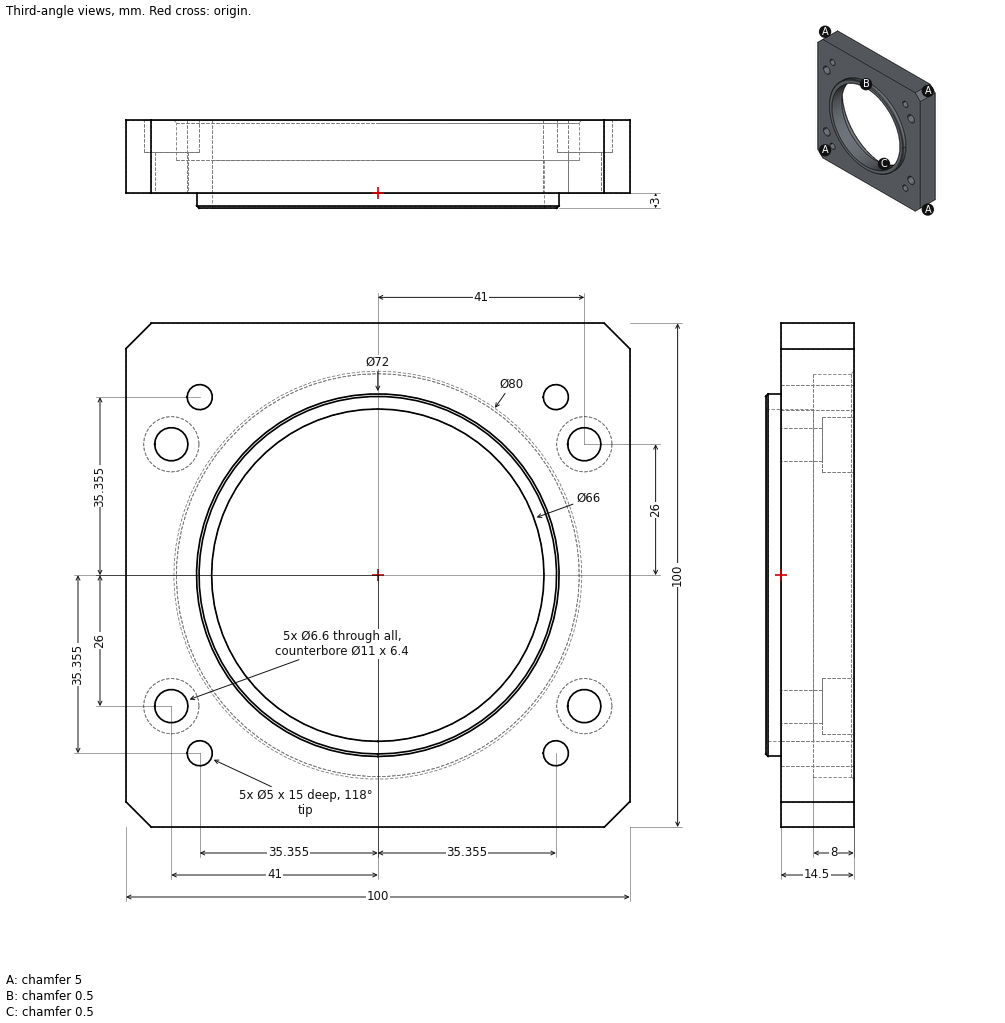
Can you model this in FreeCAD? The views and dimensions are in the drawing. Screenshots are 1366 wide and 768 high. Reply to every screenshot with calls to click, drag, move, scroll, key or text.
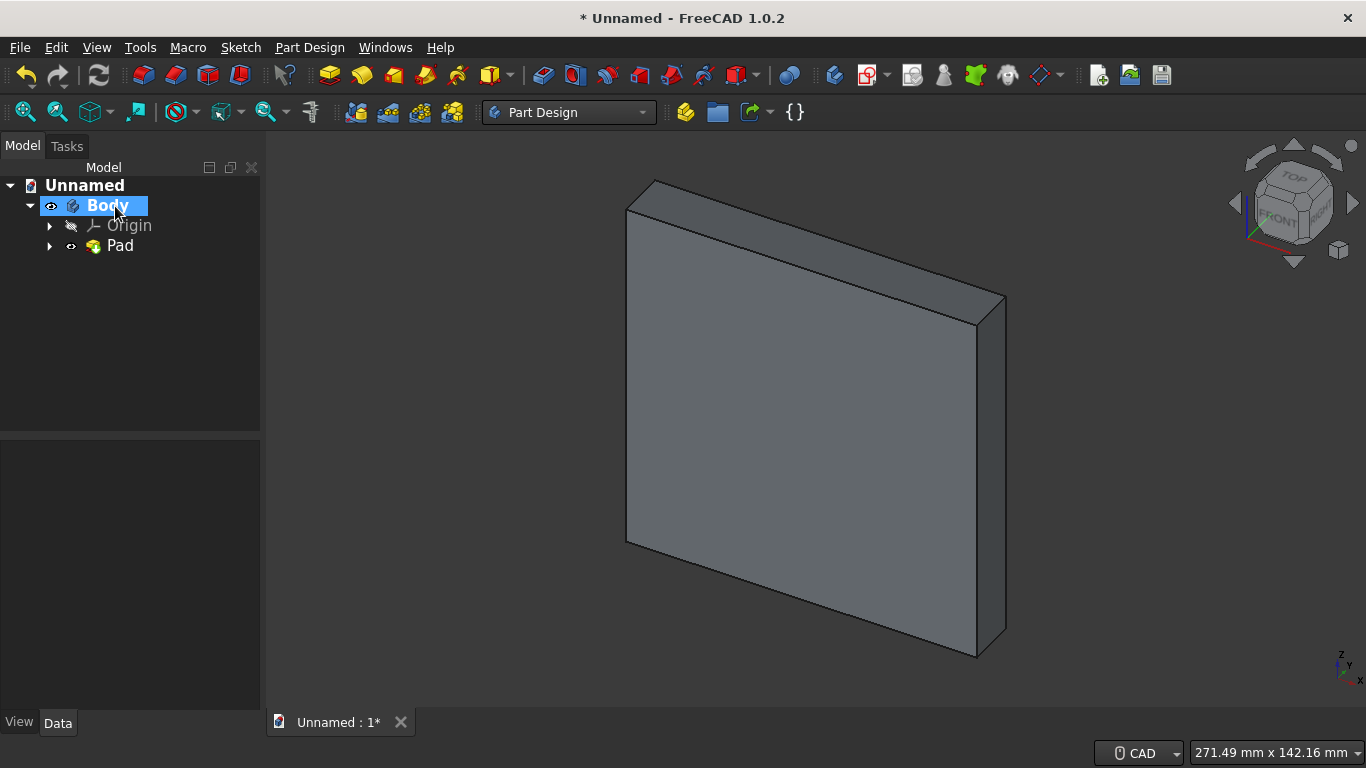
click(801, 433)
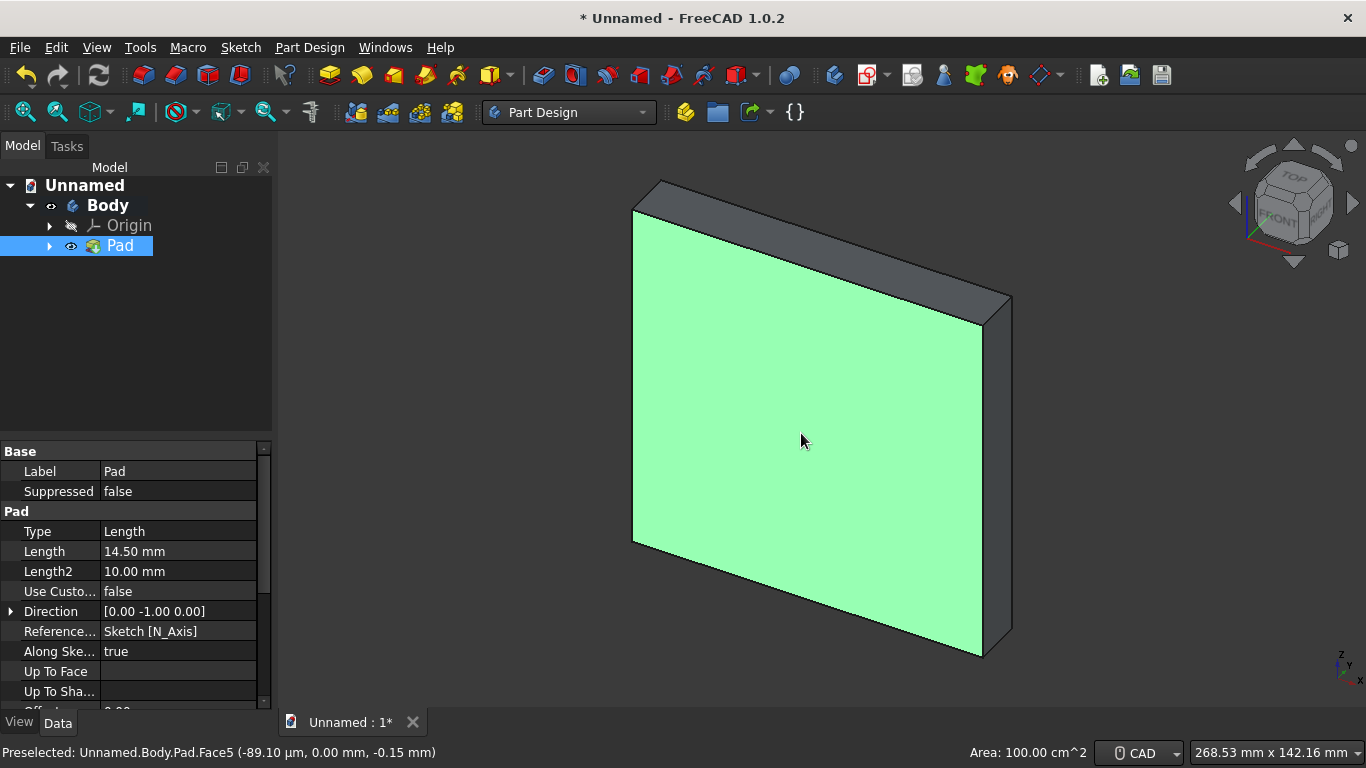
click(868, 76)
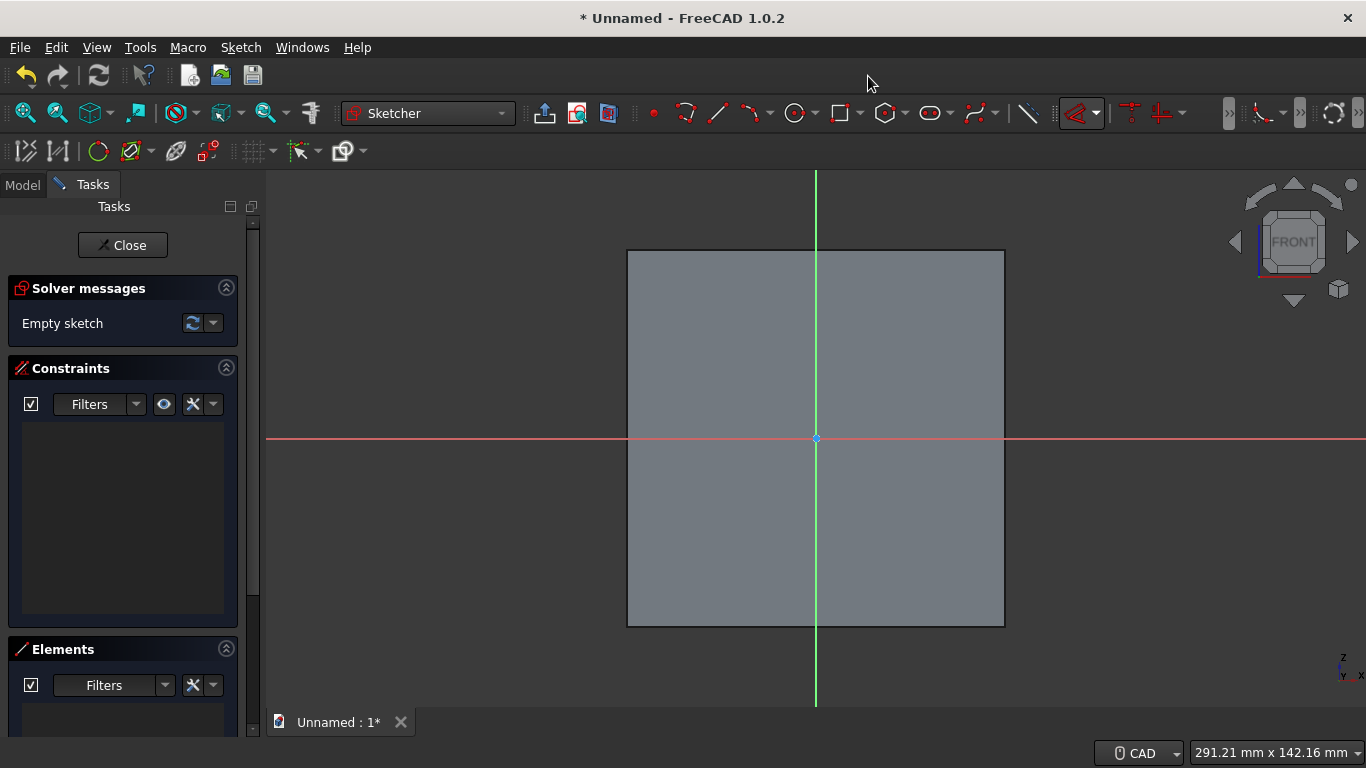
key(g)
key(c)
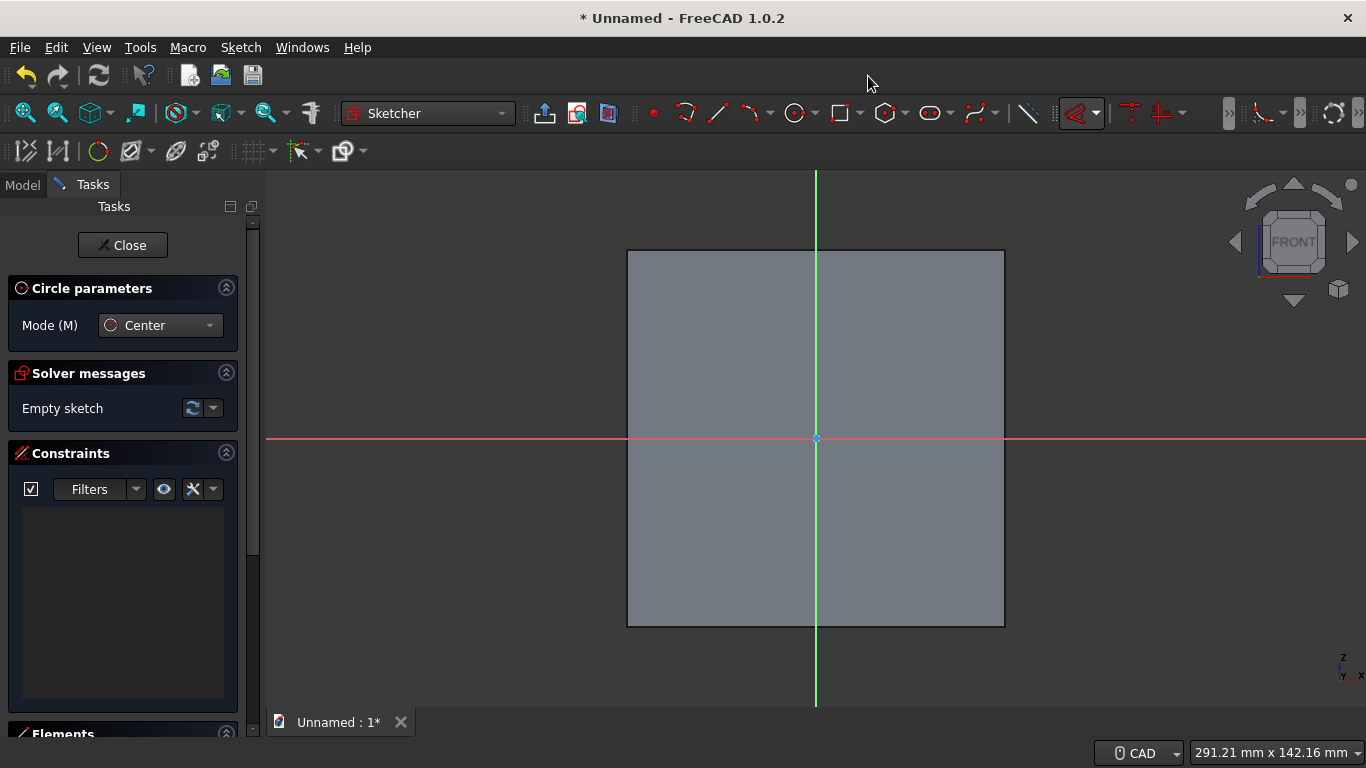
click(816, 438)
click(912, 342)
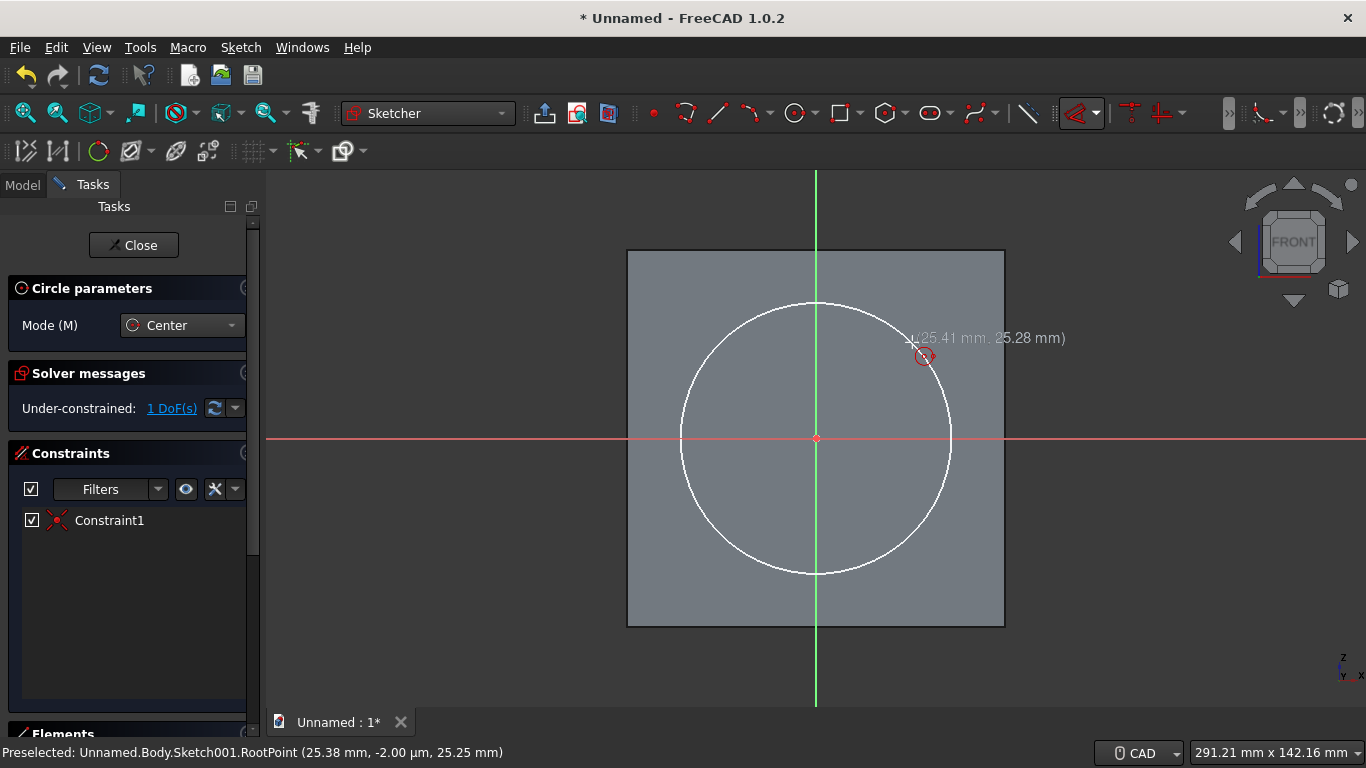
click(816, 438)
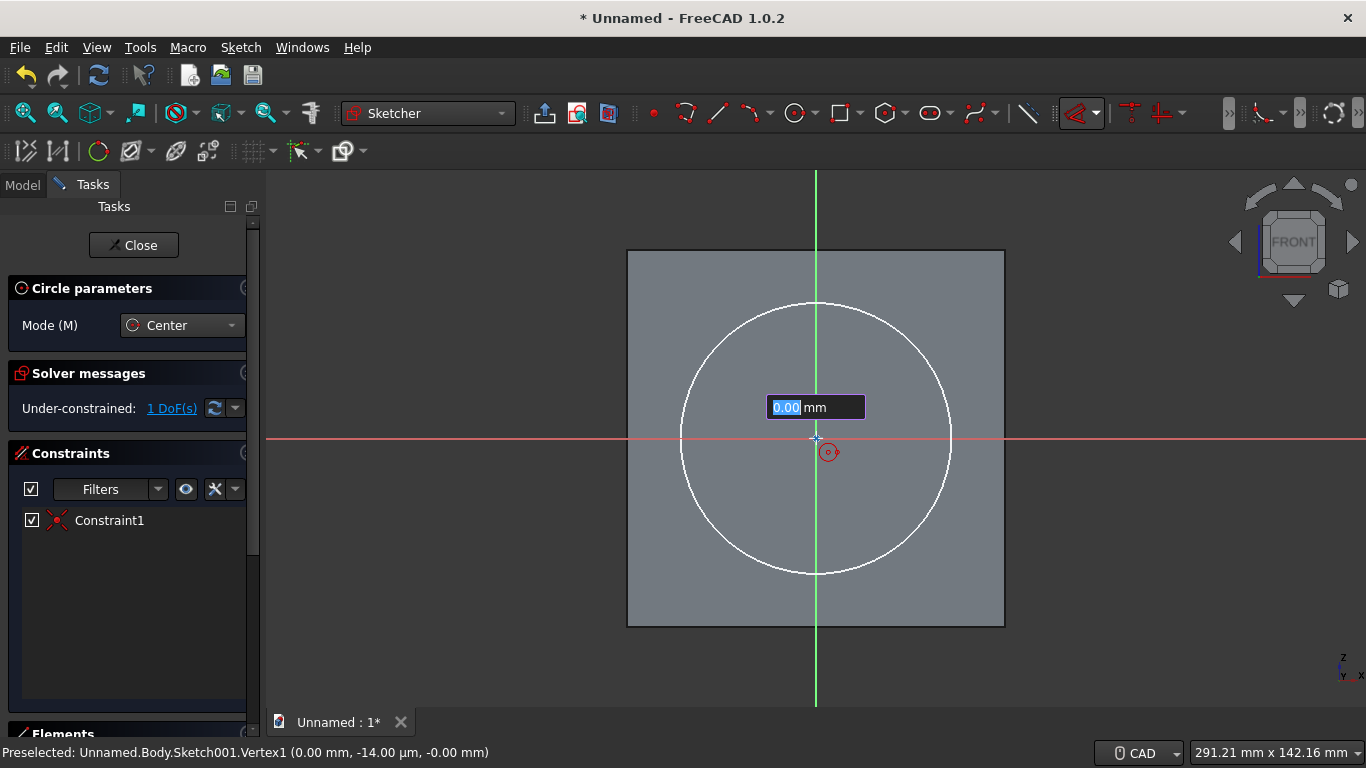
scroll(904, 350, up, 2)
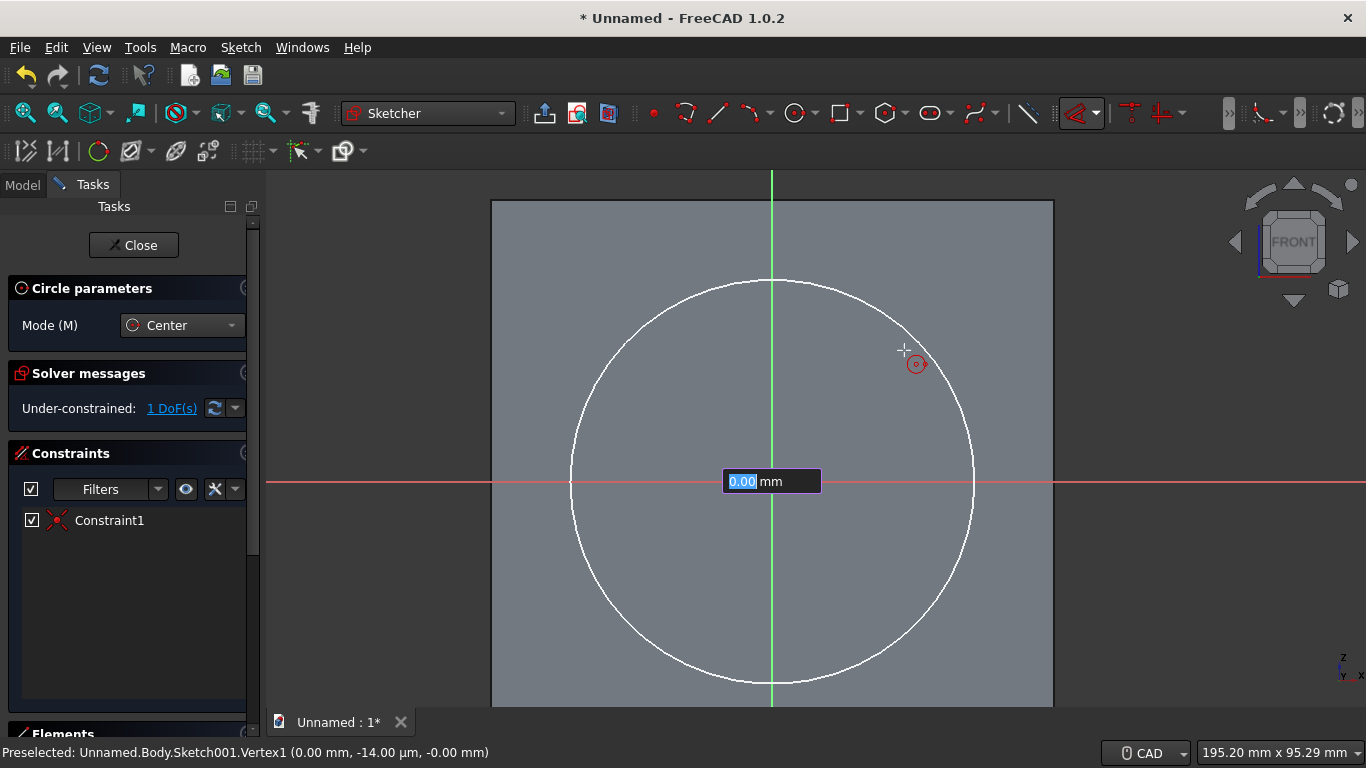
click(904, 350)
key(Escape)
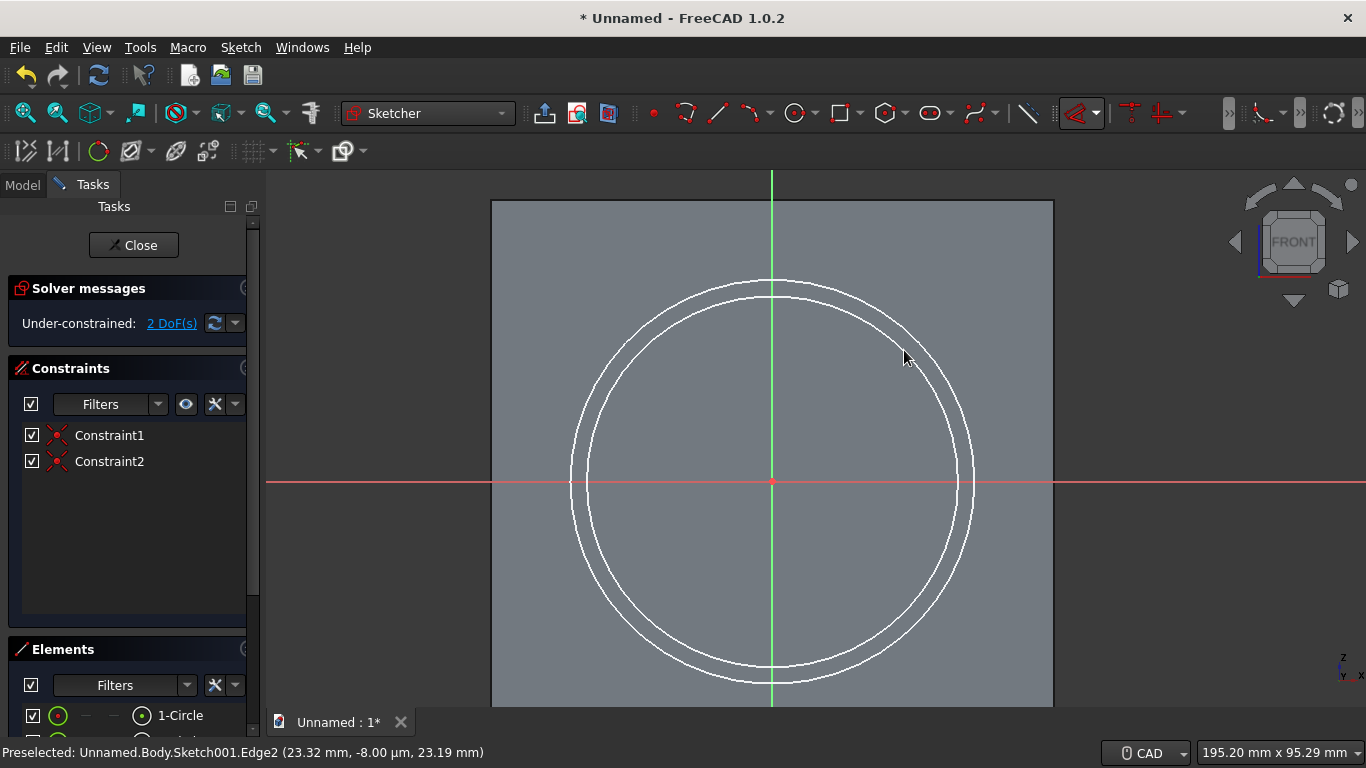
key(d)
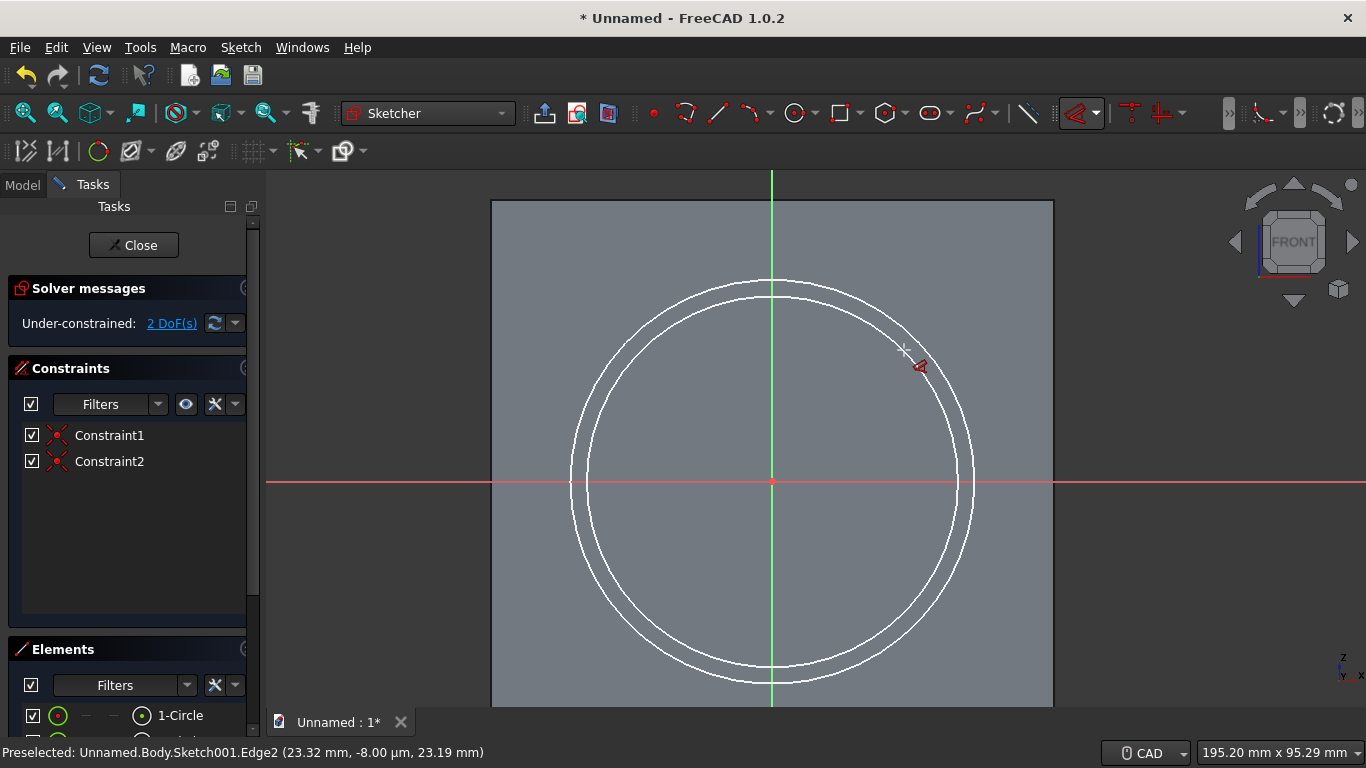
click(915, 339)
click(938, 316)